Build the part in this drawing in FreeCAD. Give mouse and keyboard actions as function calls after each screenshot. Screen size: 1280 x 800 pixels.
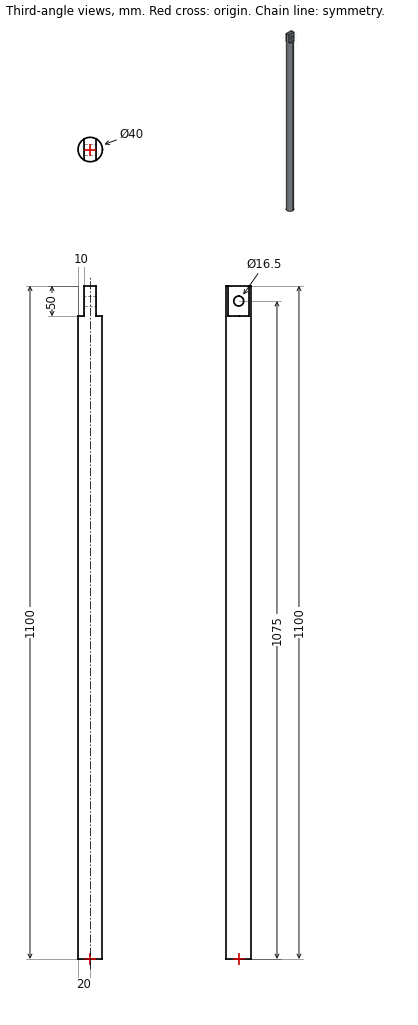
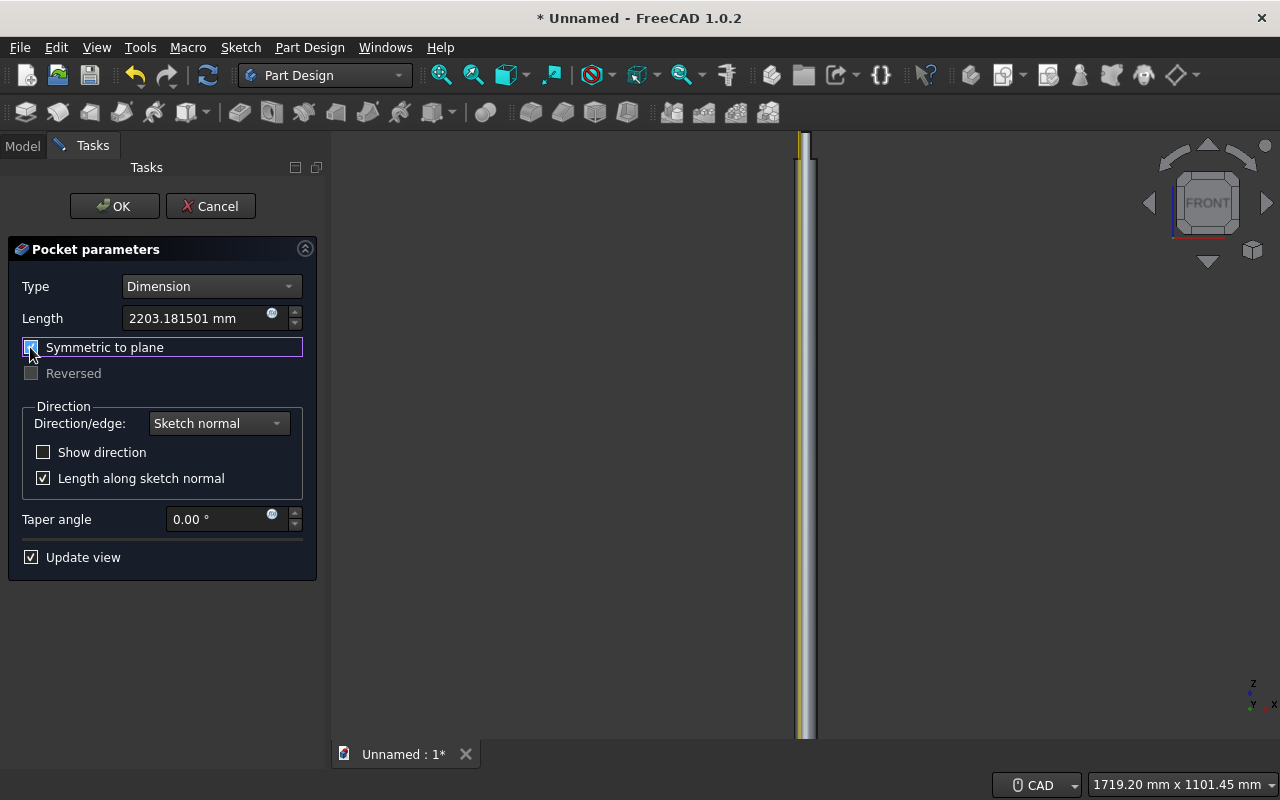
click(115, 206)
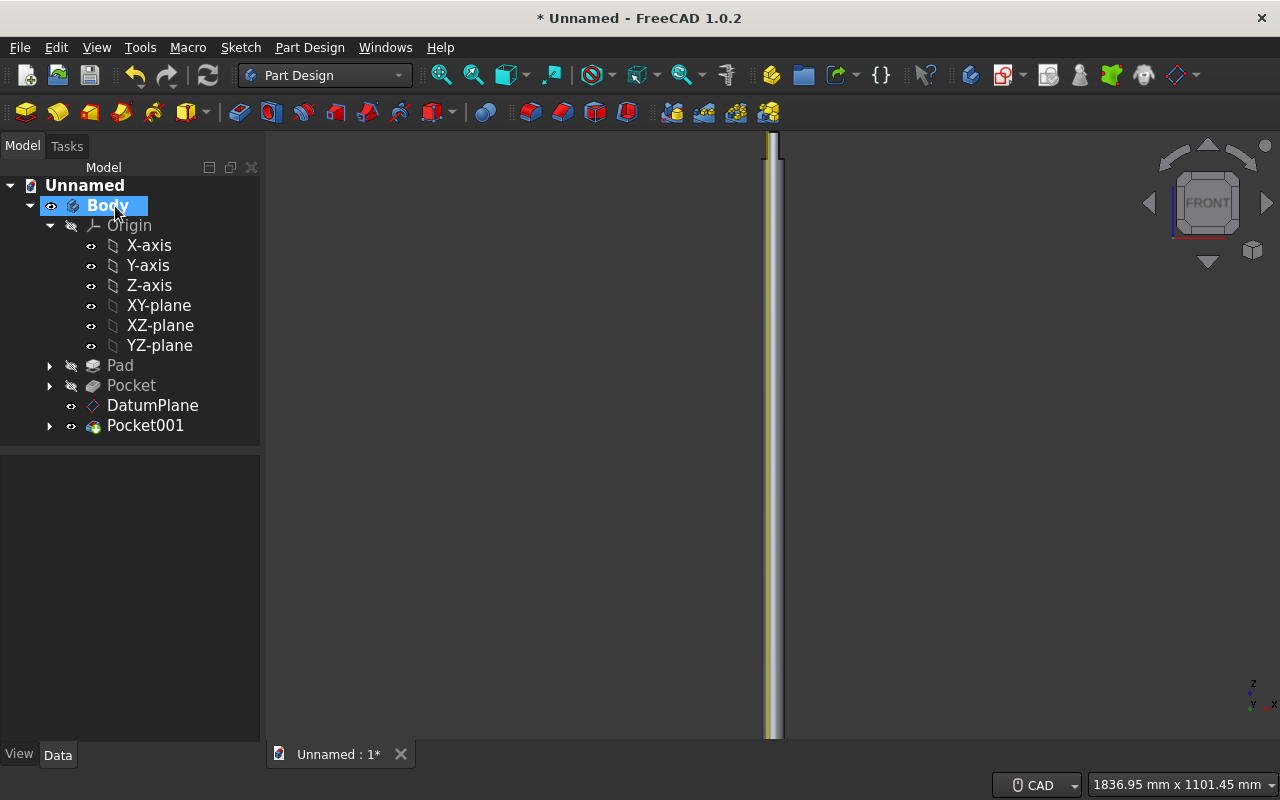
click(116, 406)
key(space)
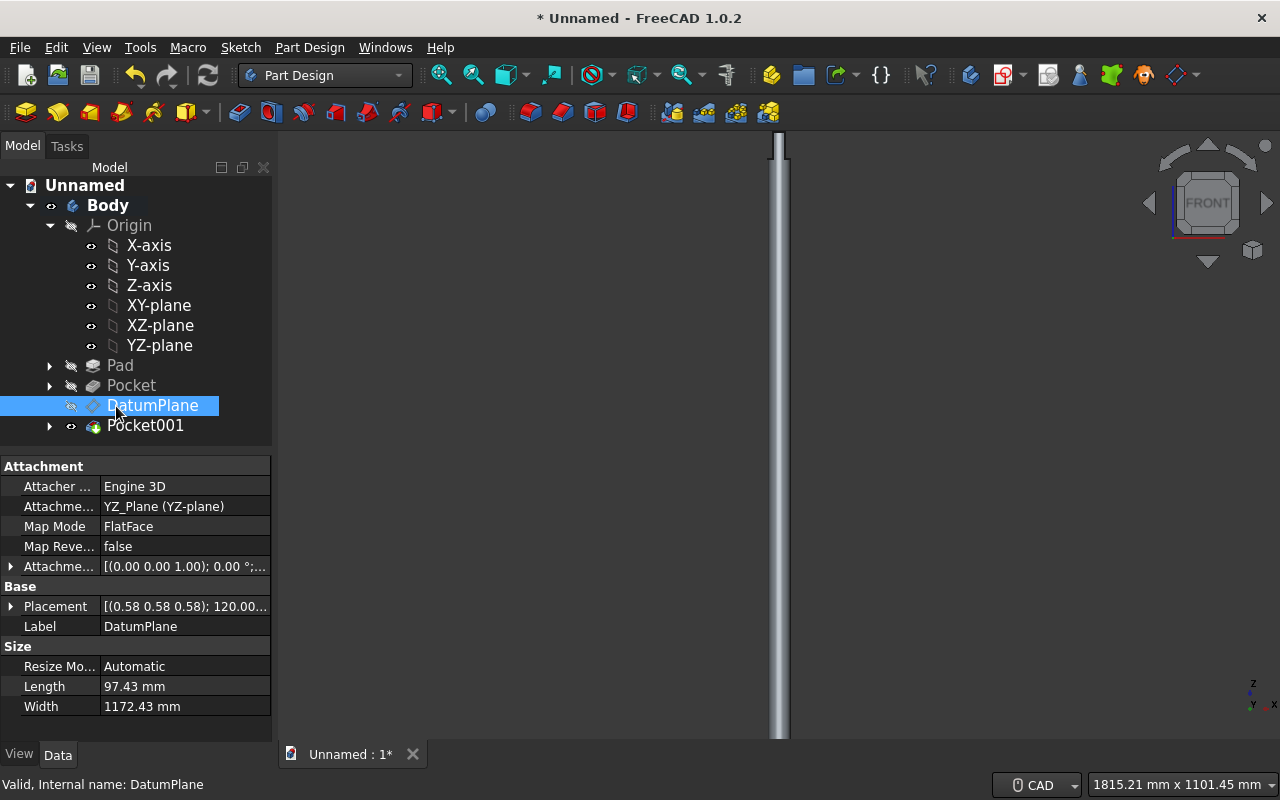
key(0)